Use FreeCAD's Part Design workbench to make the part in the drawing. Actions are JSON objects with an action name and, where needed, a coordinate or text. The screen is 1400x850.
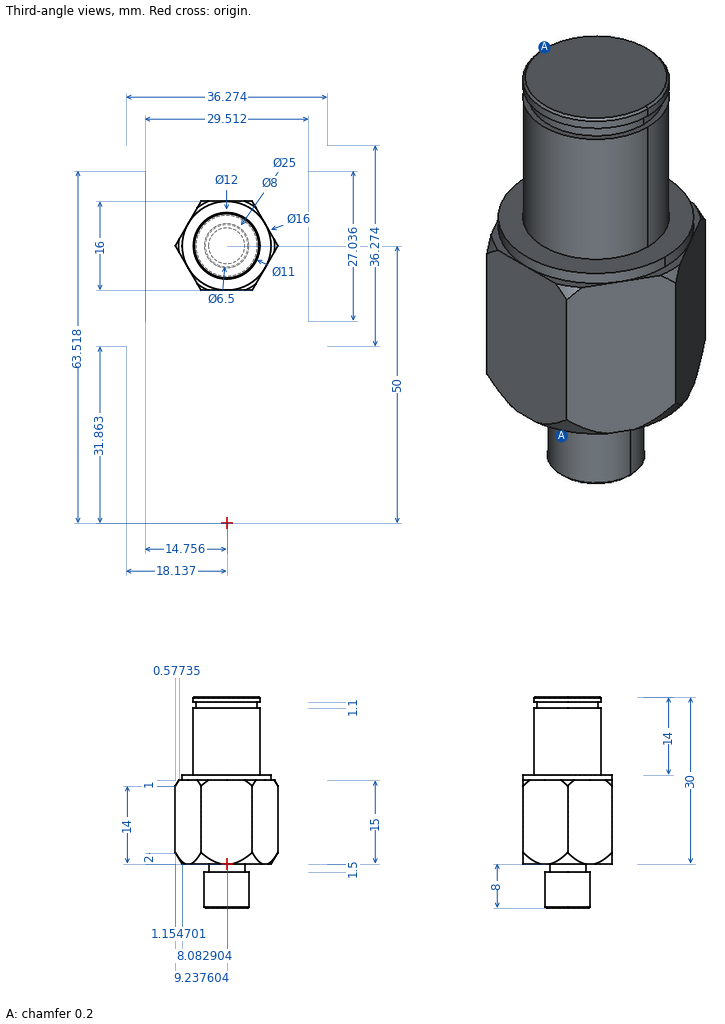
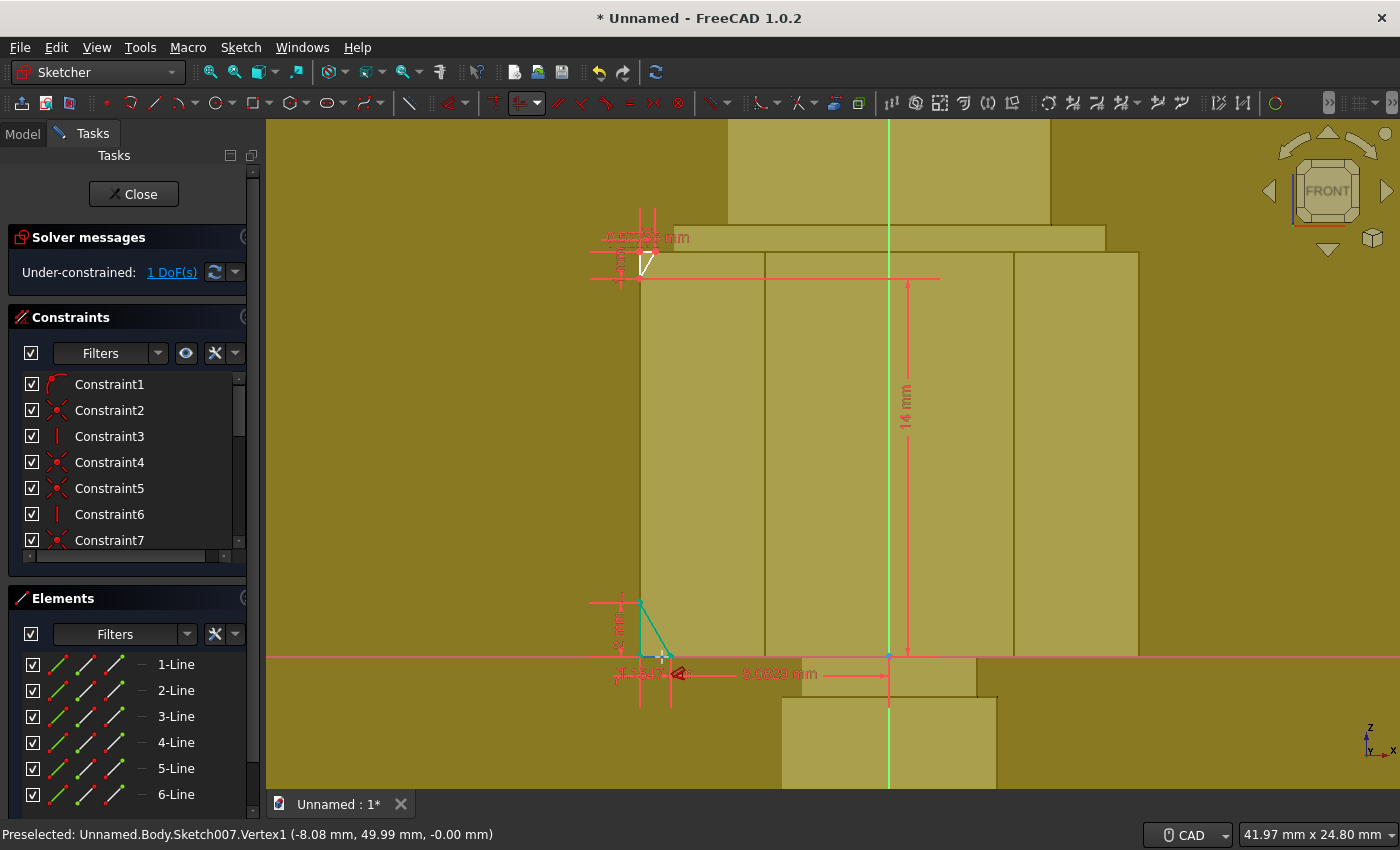
{"action": "left_click", "coordinate": [640, 279]}
{"action": "left_click", "coordinate": [852, 691]}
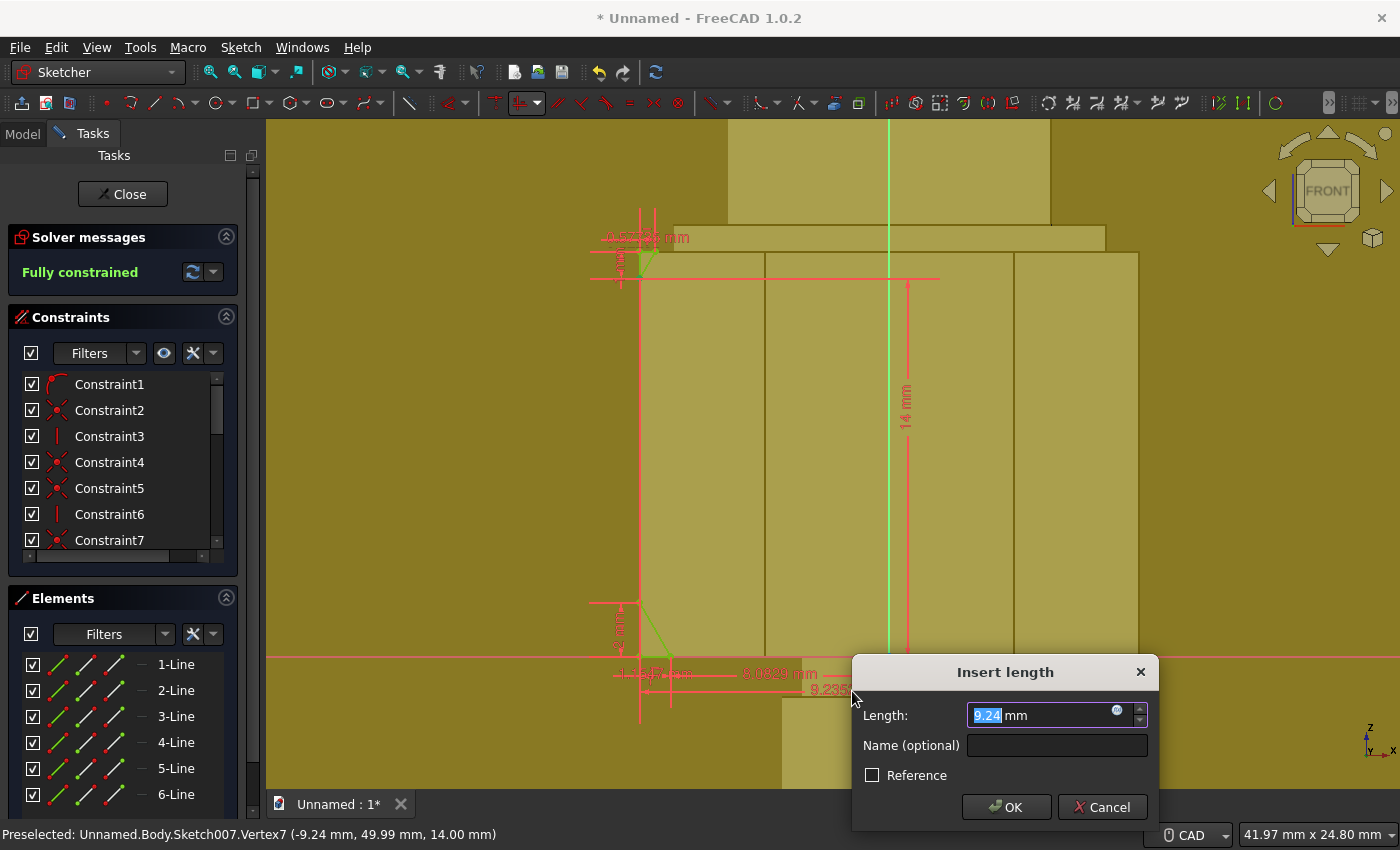
{"action": "type", "text": "9.237604"}
{"action": "key", "text": "Return"}
{"action": "key", "text": "Escape"}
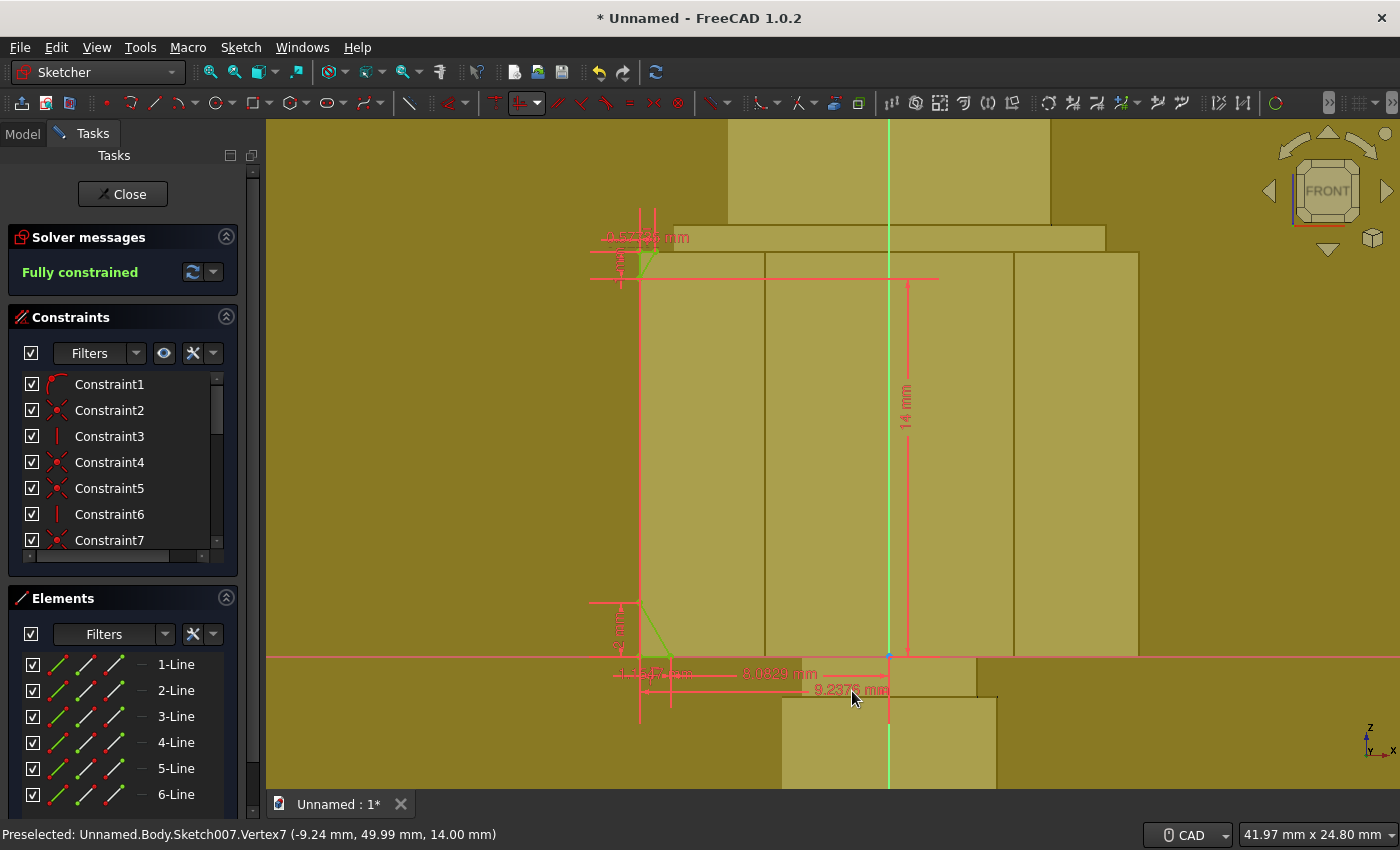
{"action": "left_click", "coordinate": [123, 194]}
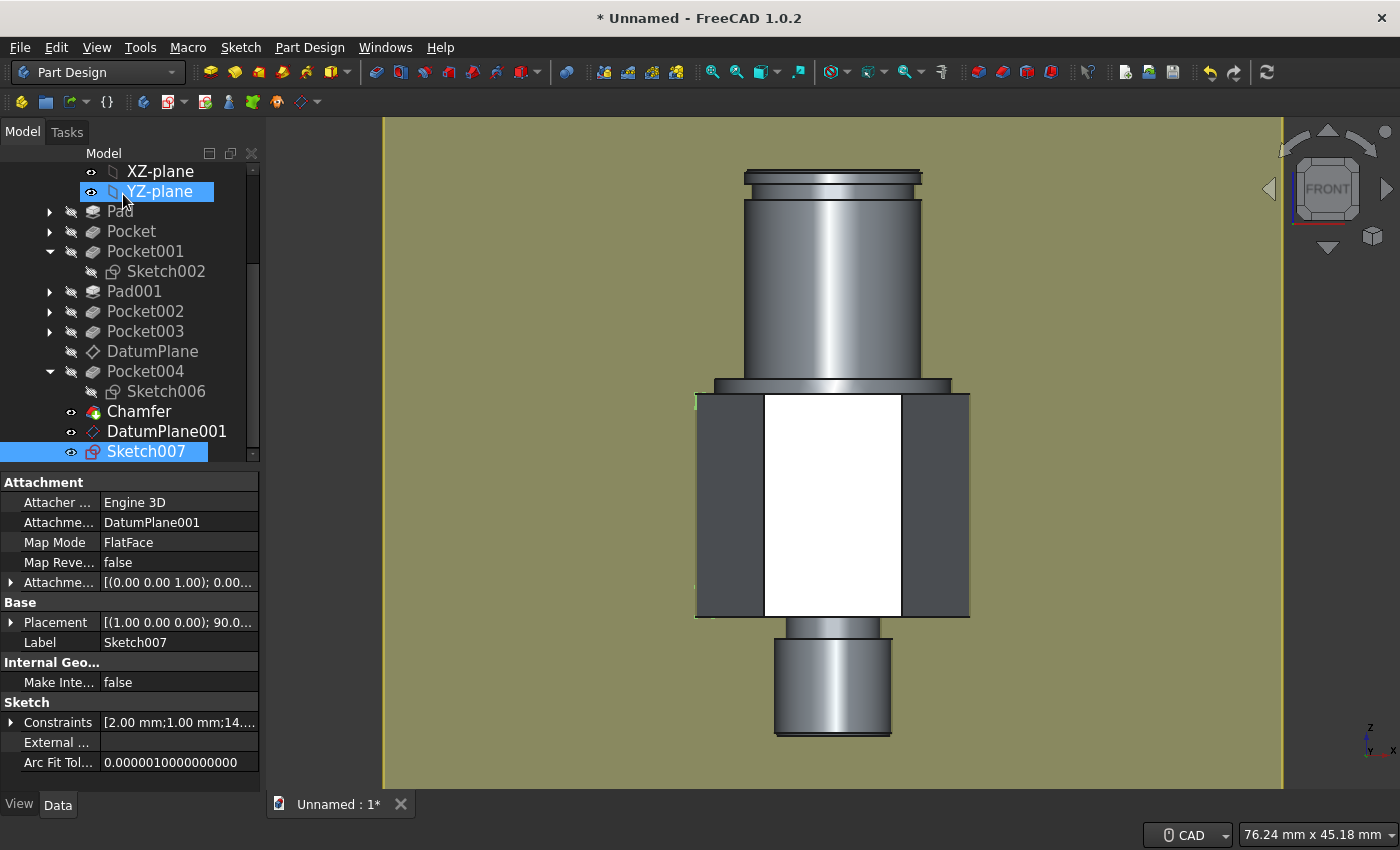
{"action": "left_click", "coordinate": [426, 72]}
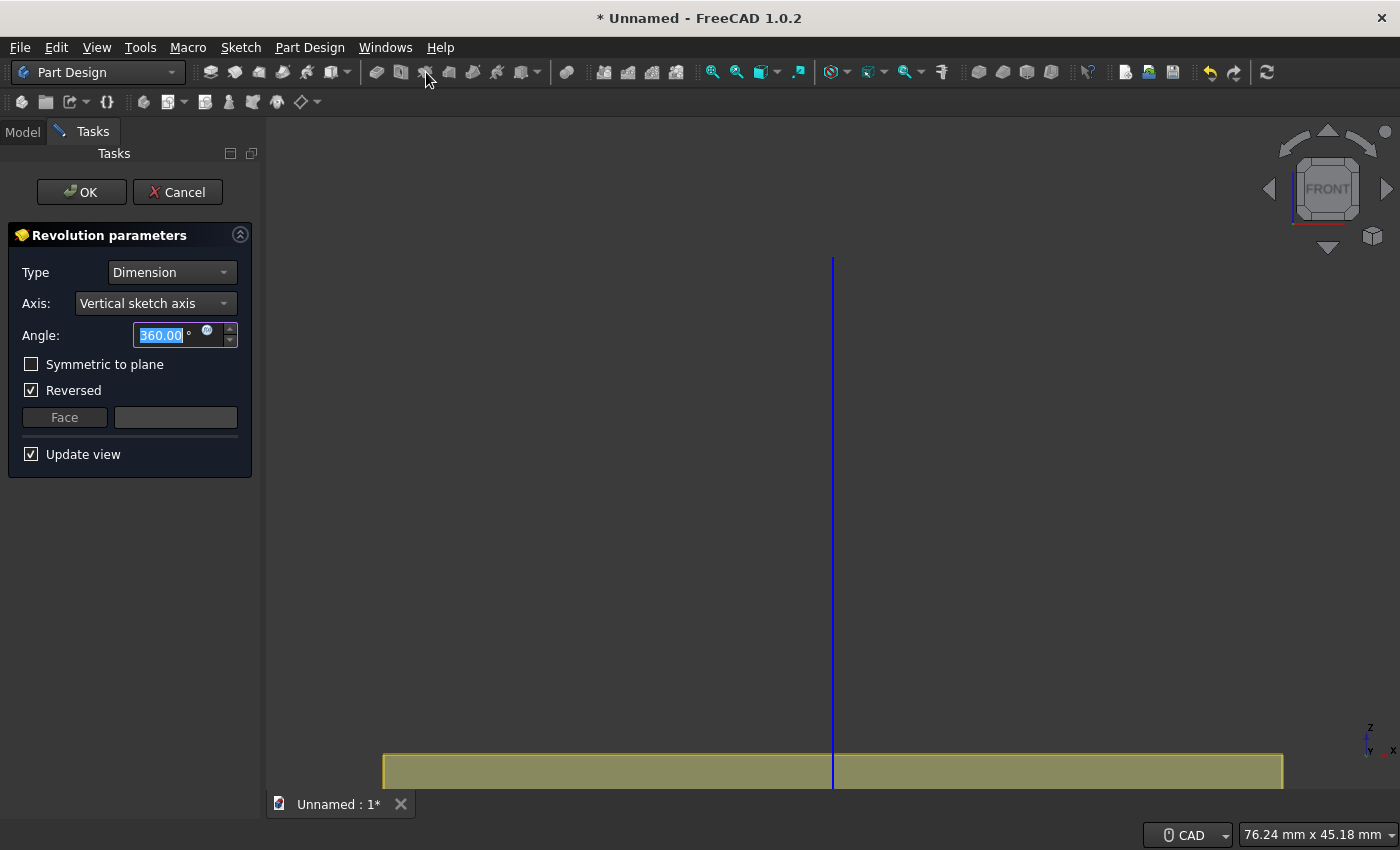
{"action": "left_click", "coordinate": [82, 192]}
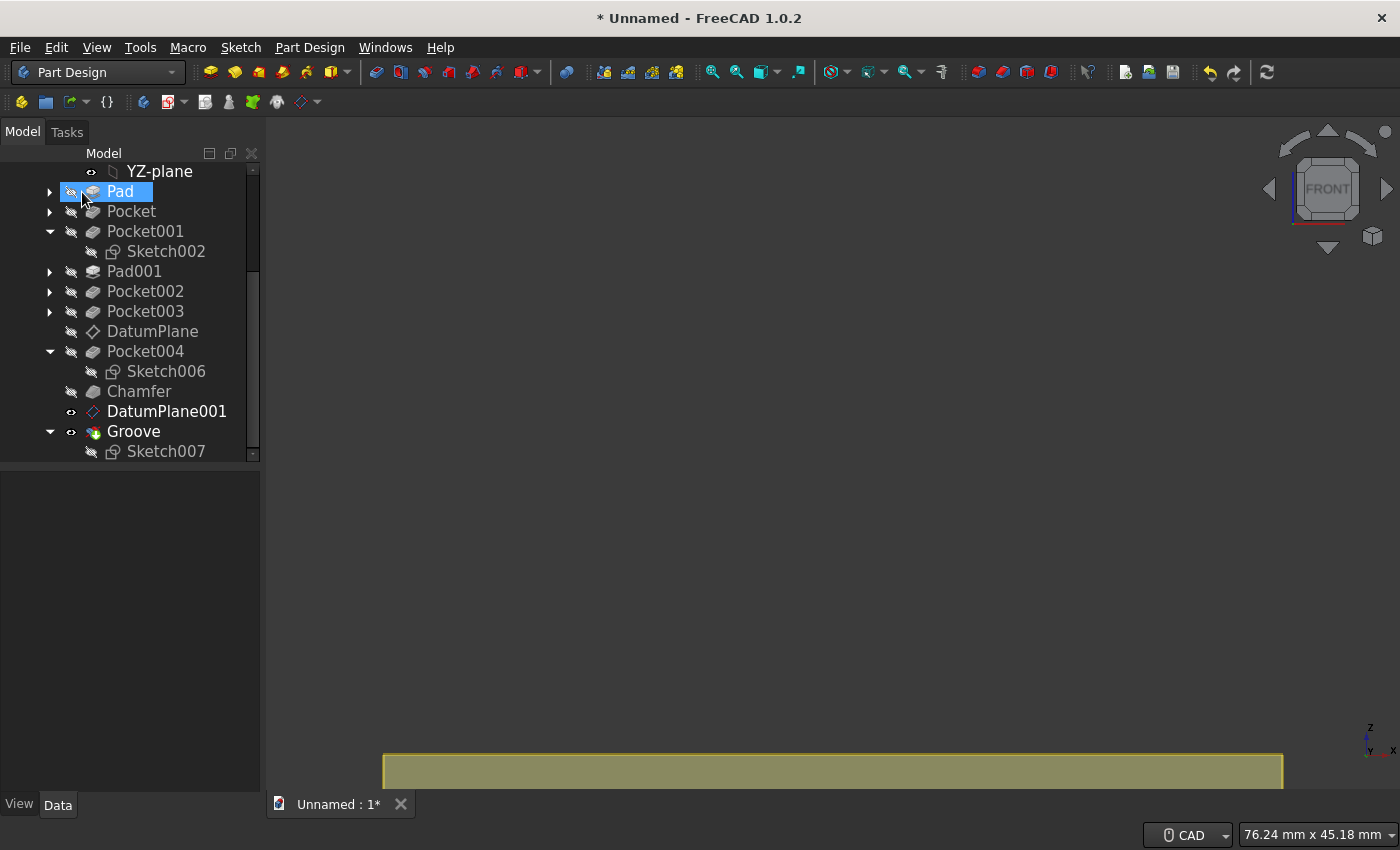
{"action": "left_click", "coordinate": [116, 412]}
{"action": "key", "text": "space"}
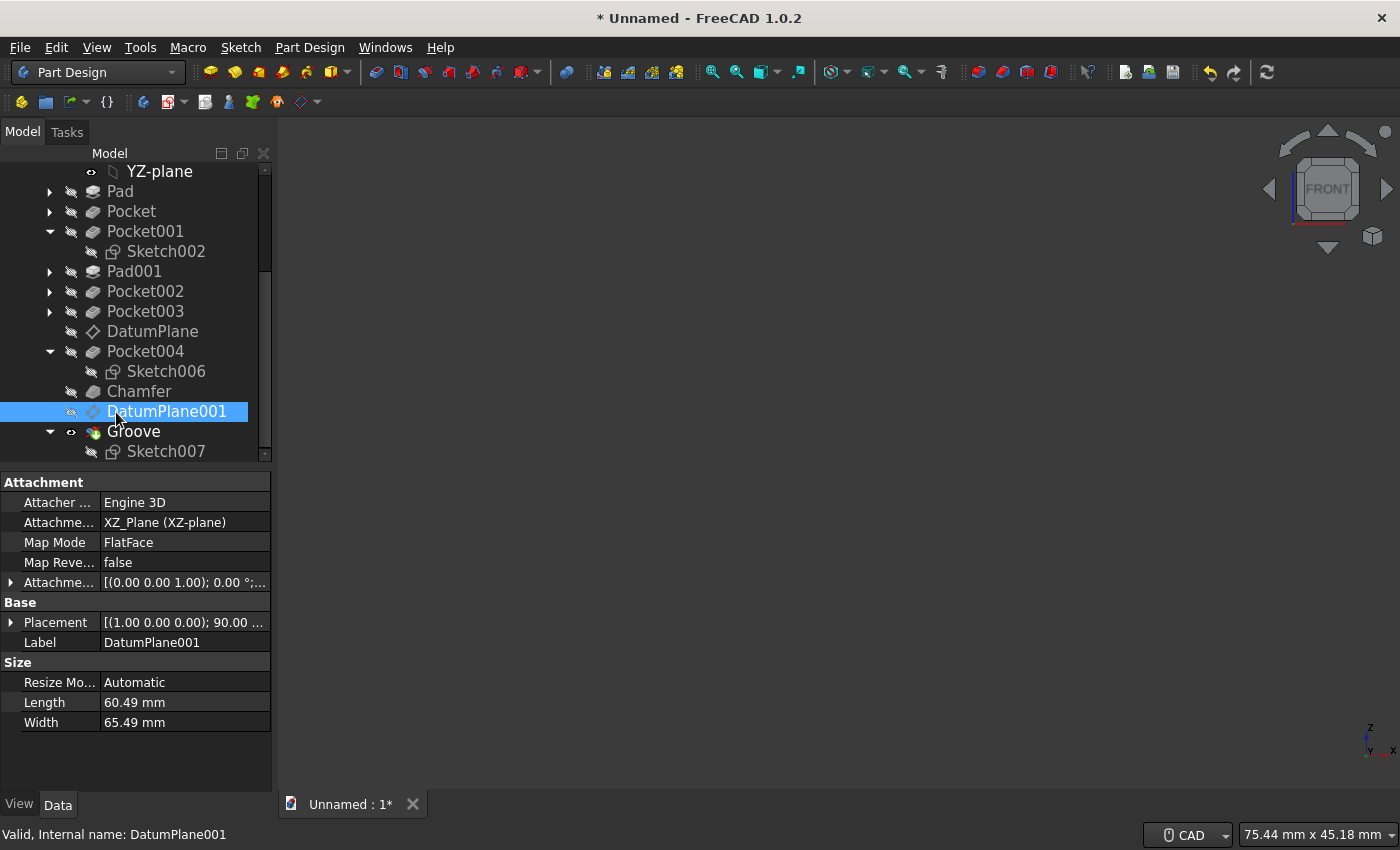
{"action": "key", "text": "0"}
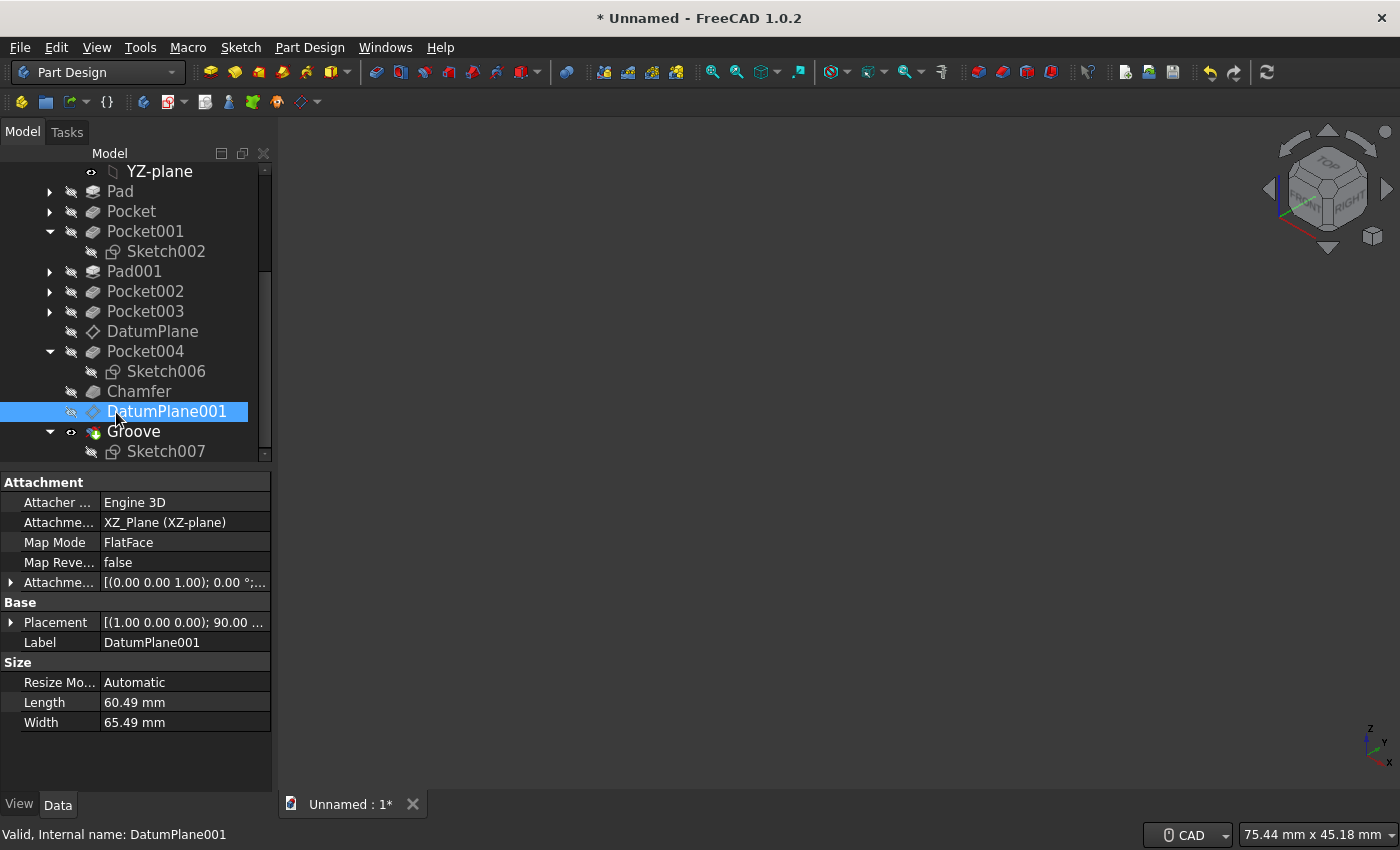
{"action": "left_click", "coordinate": [714, 72]}